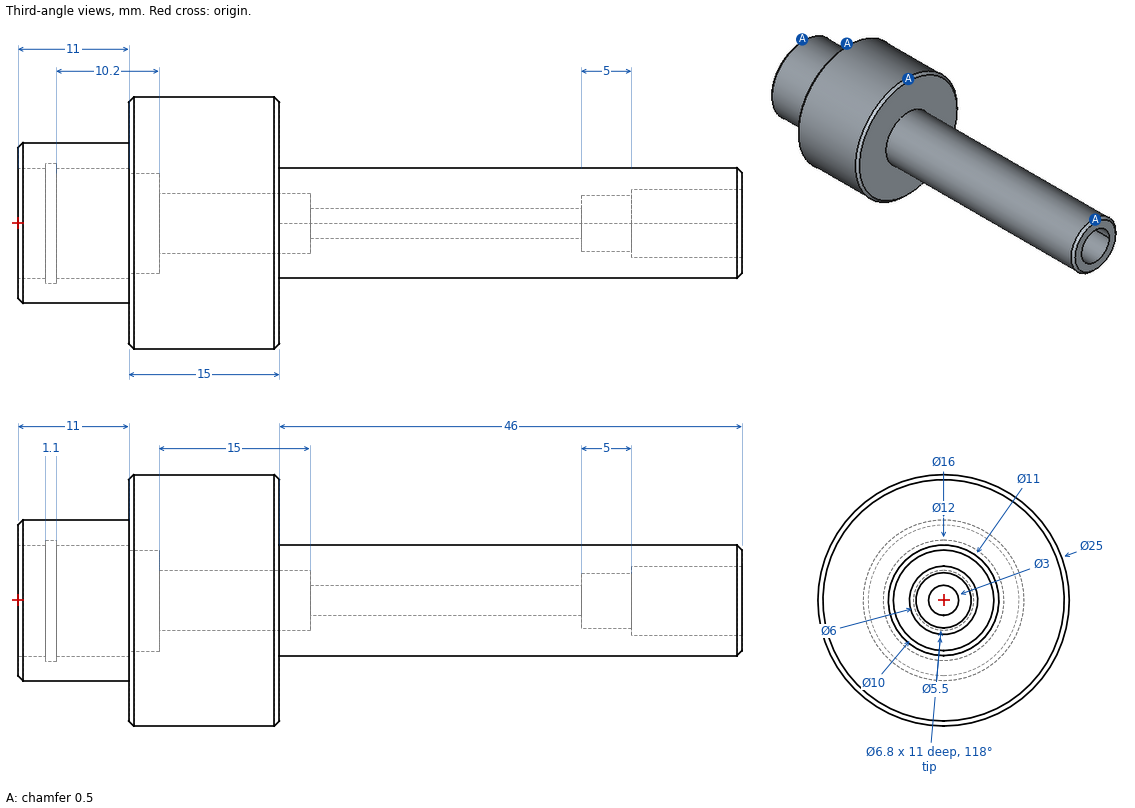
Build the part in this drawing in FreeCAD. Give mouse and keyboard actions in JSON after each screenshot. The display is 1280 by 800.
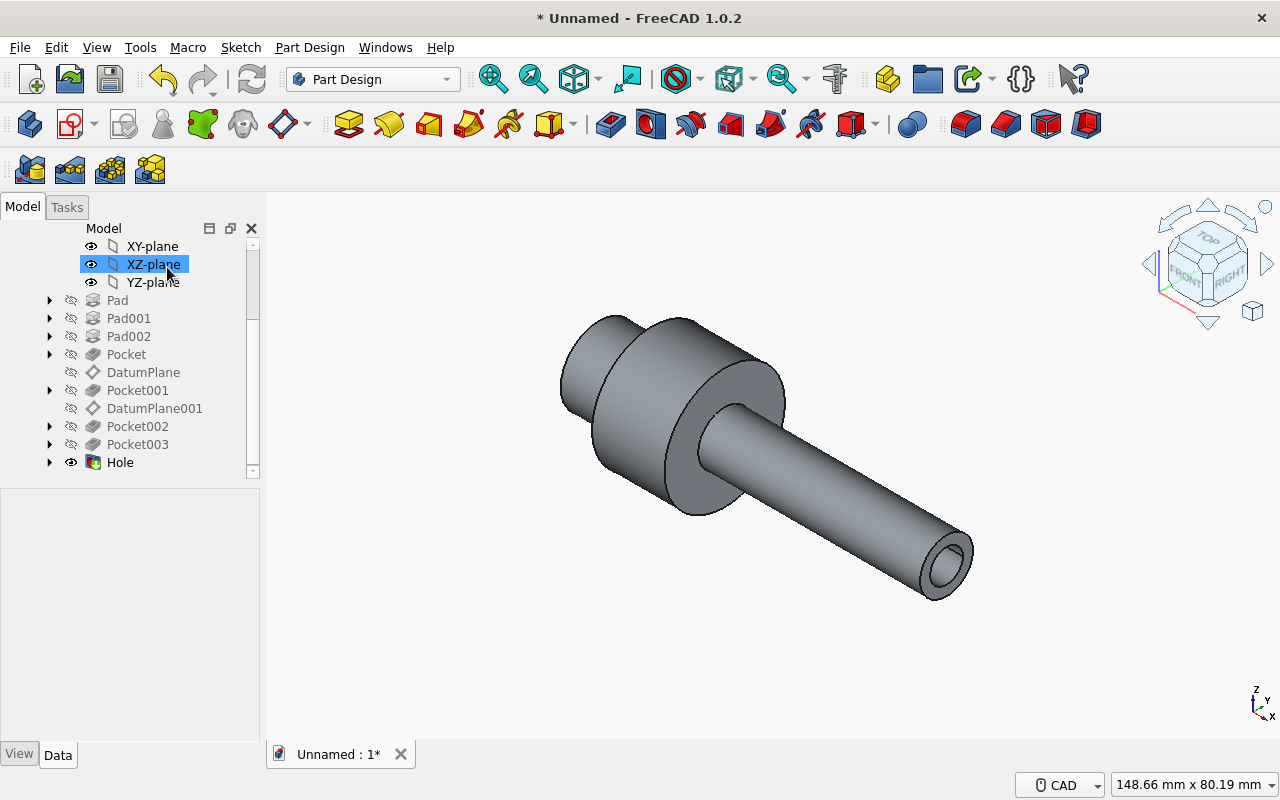
{"action": "scroll", "coordinate": [160, 350], "scroll_direction": "down", "scroll_amount": 3}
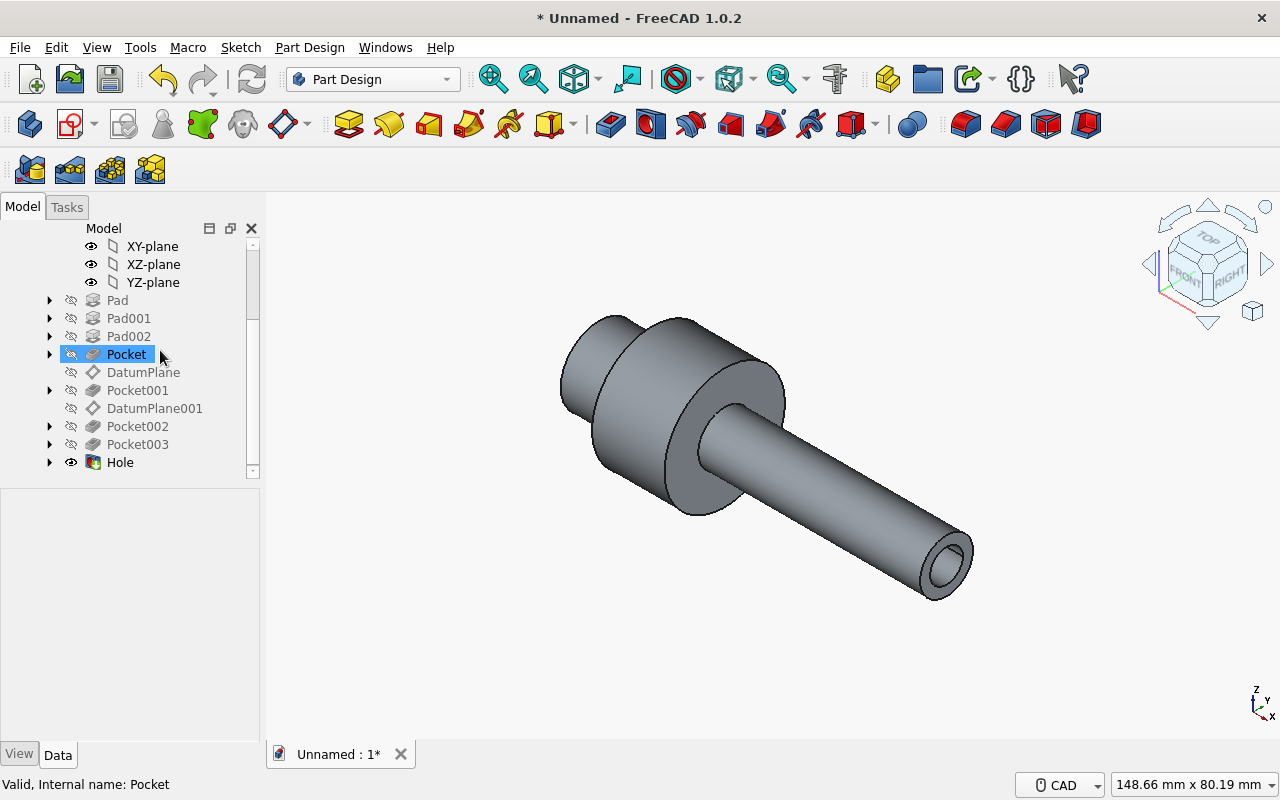
{"action": "scroll", "coordinate": [160, 350], "scroll_direction": "up", "scroll_amount": 15}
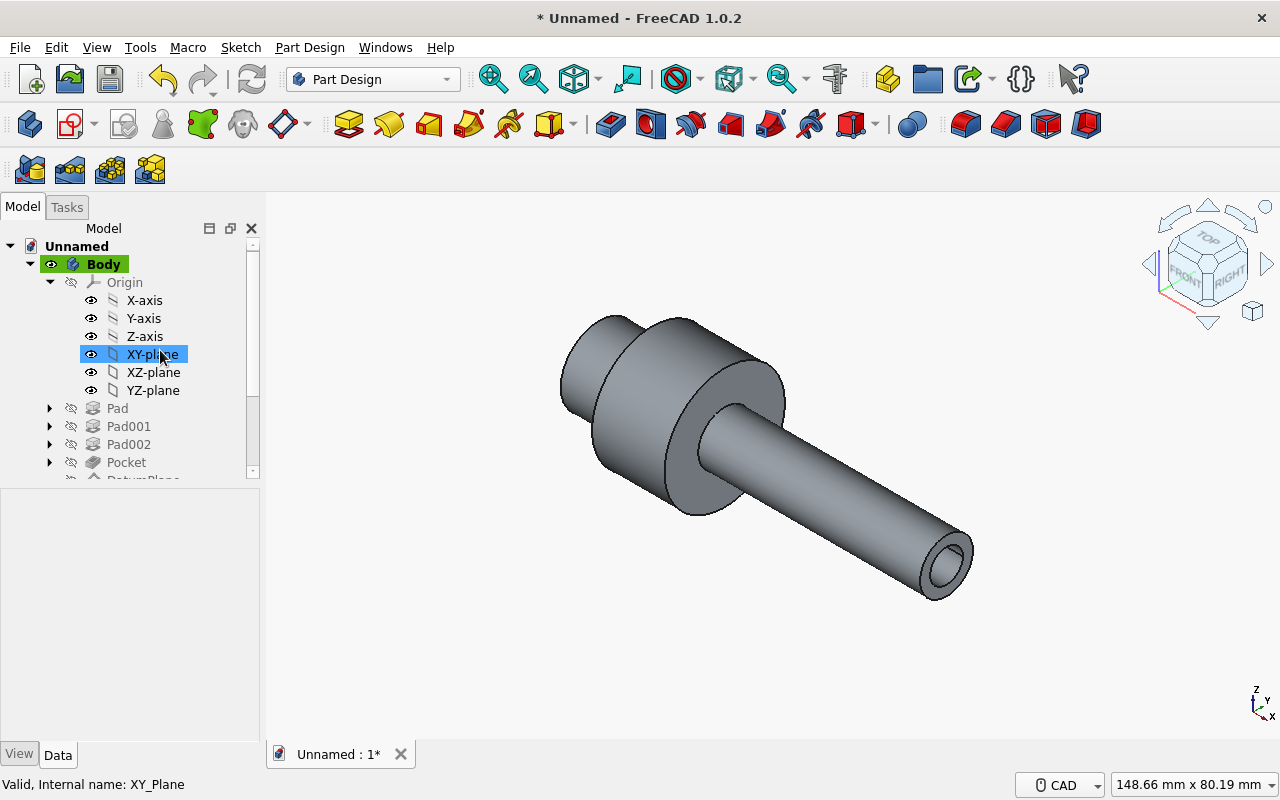
{"action": "left_click", "coordinate": [136, 390]}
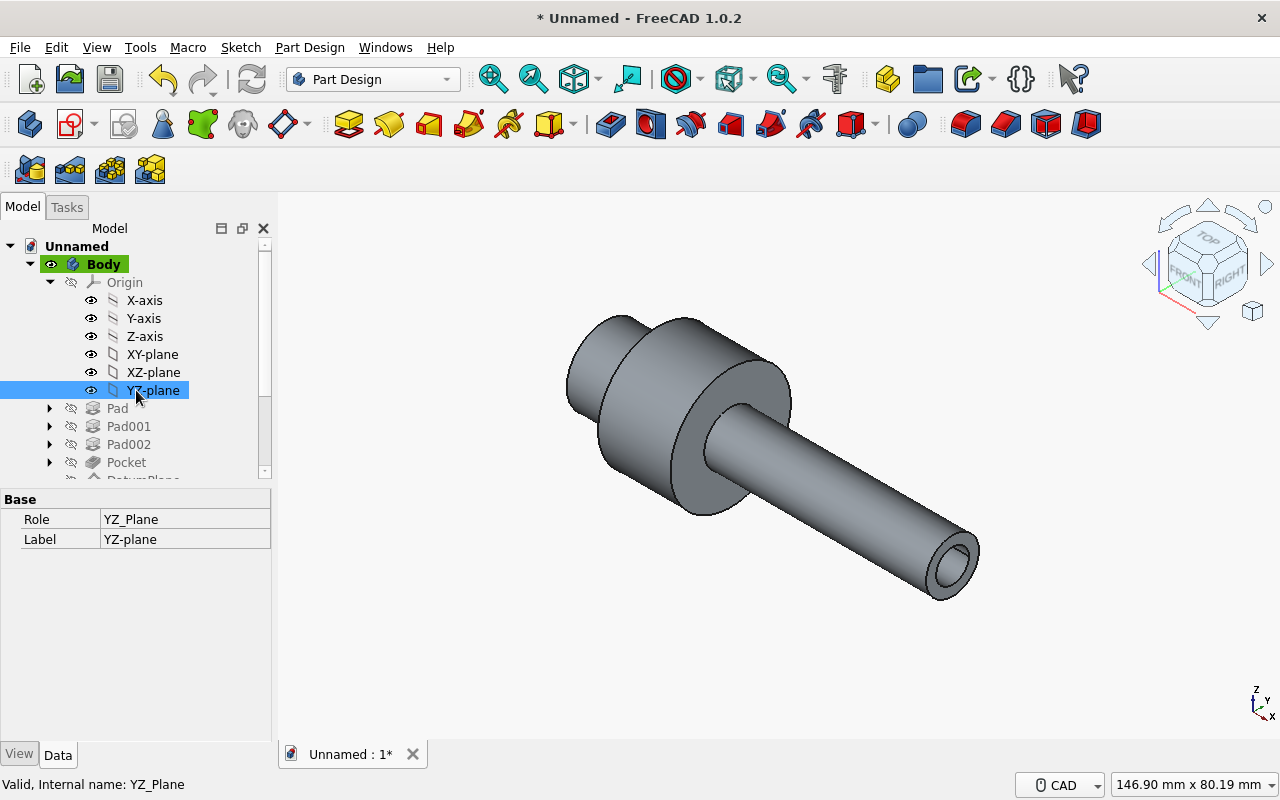
{"action": "left_click", "coordinate": [284, 124]}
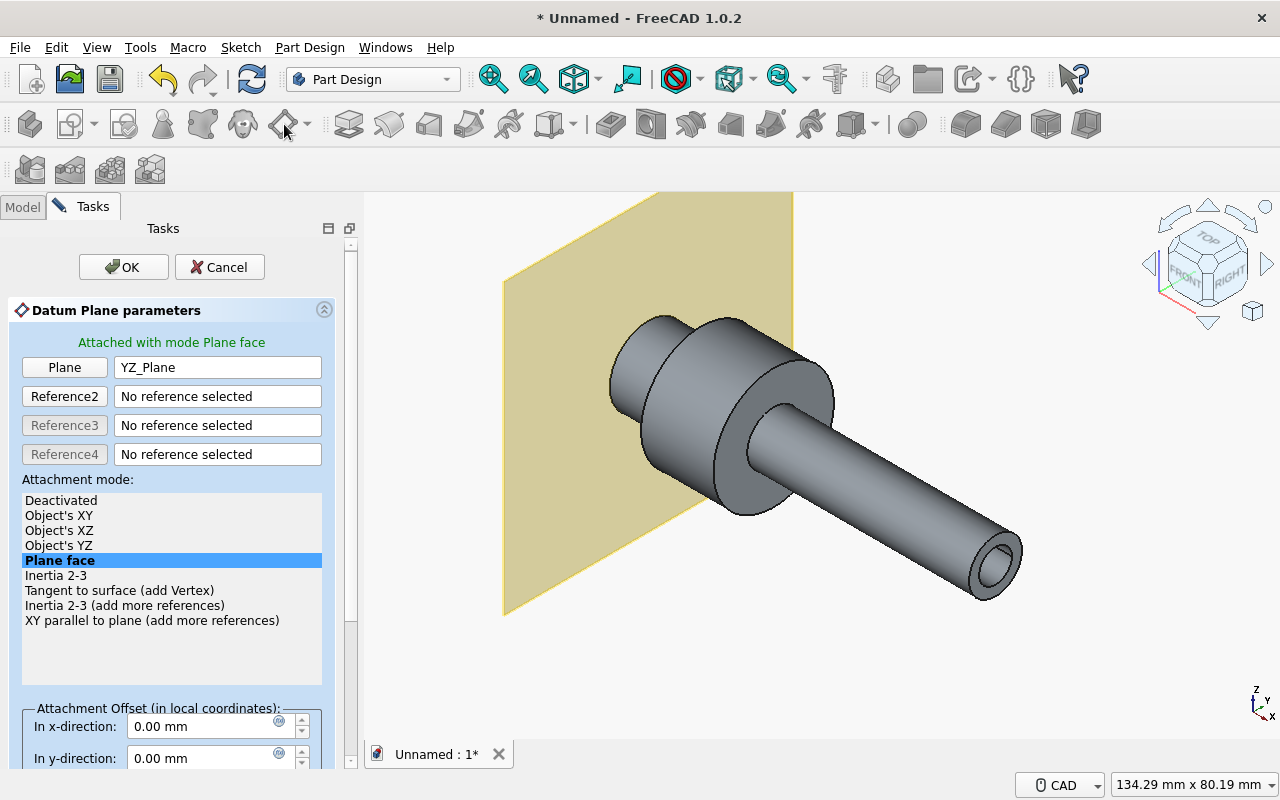
{"action": "scroll", "coordinate": [351, 503], "scroll_direction": "down", "scroll_amount": 2}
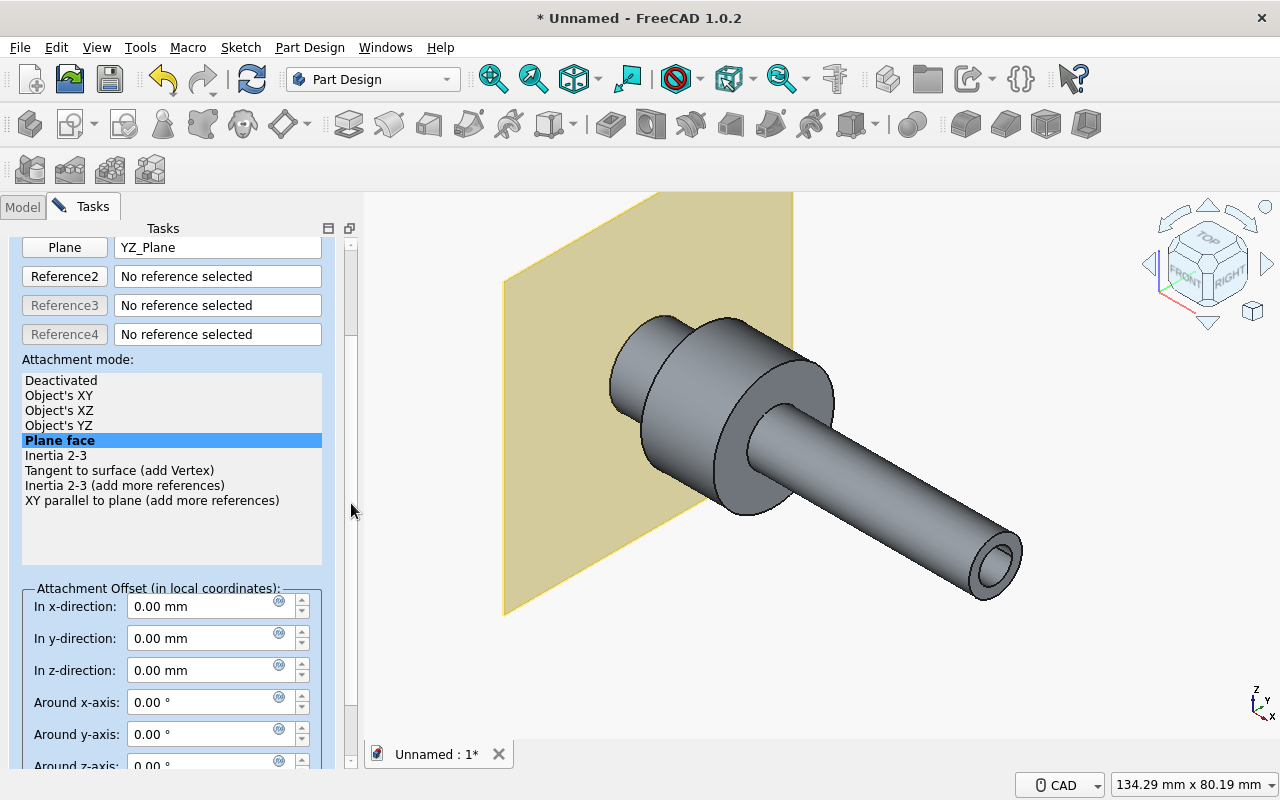
{"action": "triple_click", "coordinate": [210, 670]}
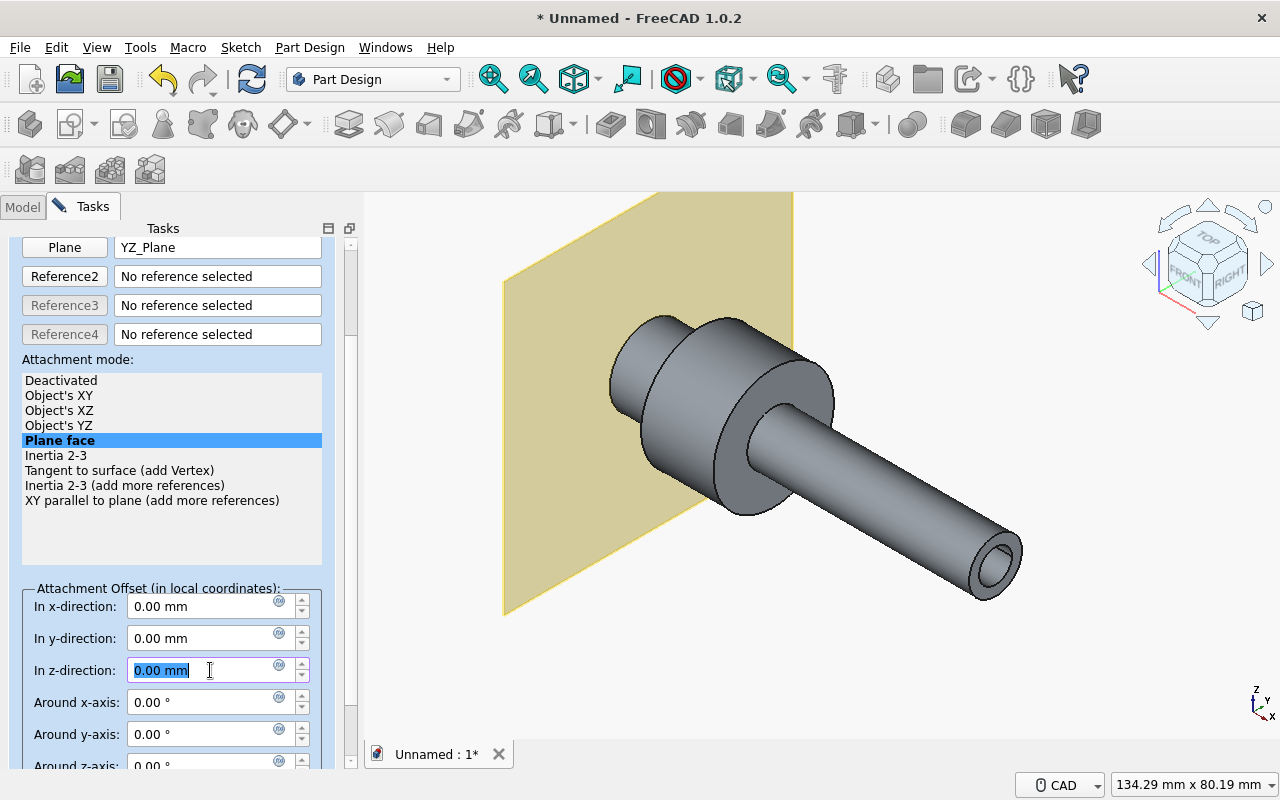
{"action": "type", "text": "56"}
{"action": "key", "text": "Tab"}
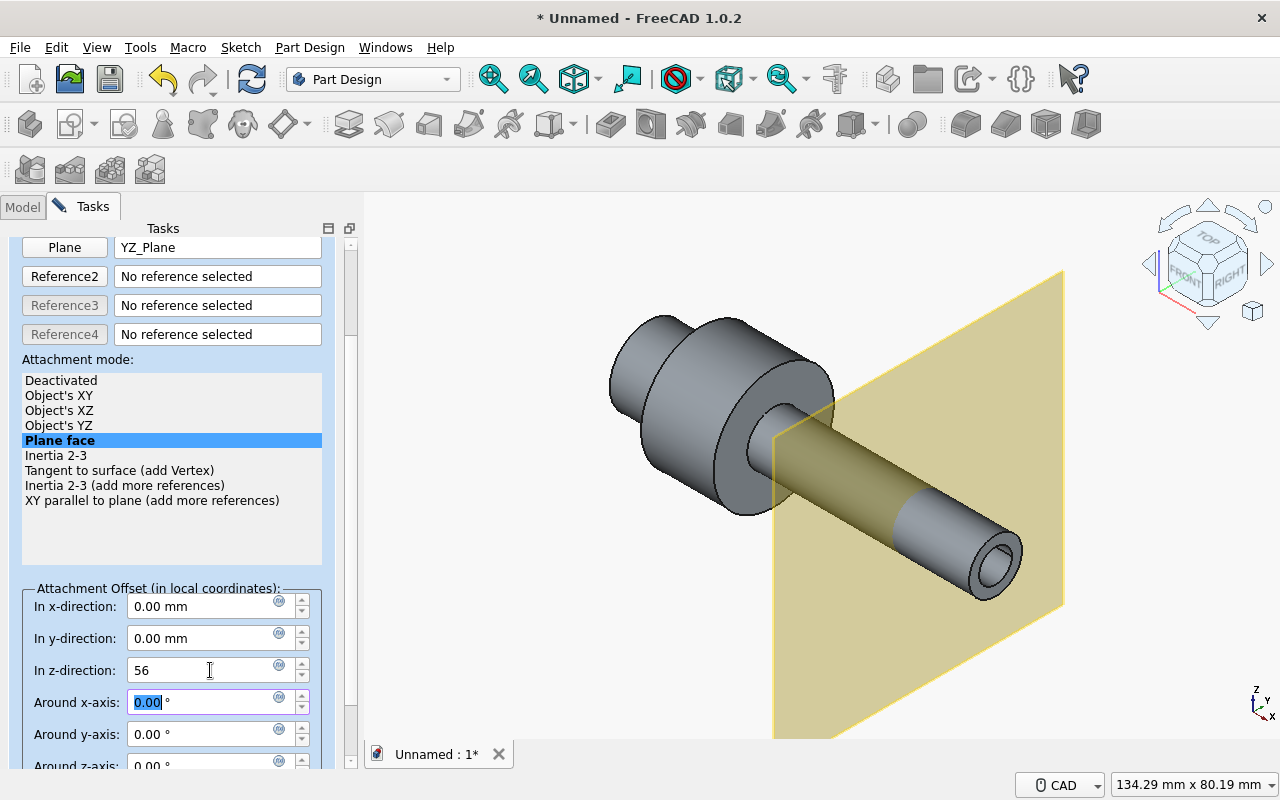
{"action": "scroll", "coordinate": [351, 503], "scroll_direction": "up", "scroll_amount": 3}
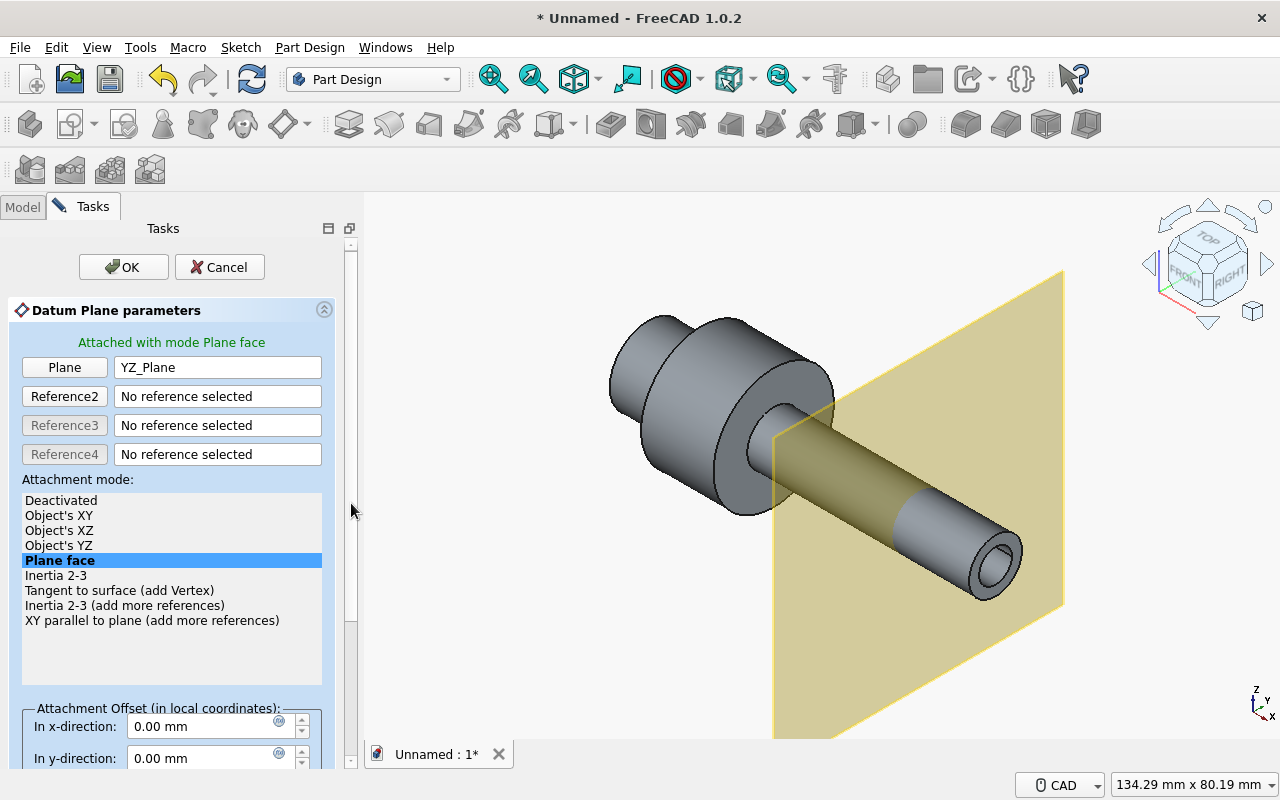
{"action": "left_click", "coordinate": [124, 267]}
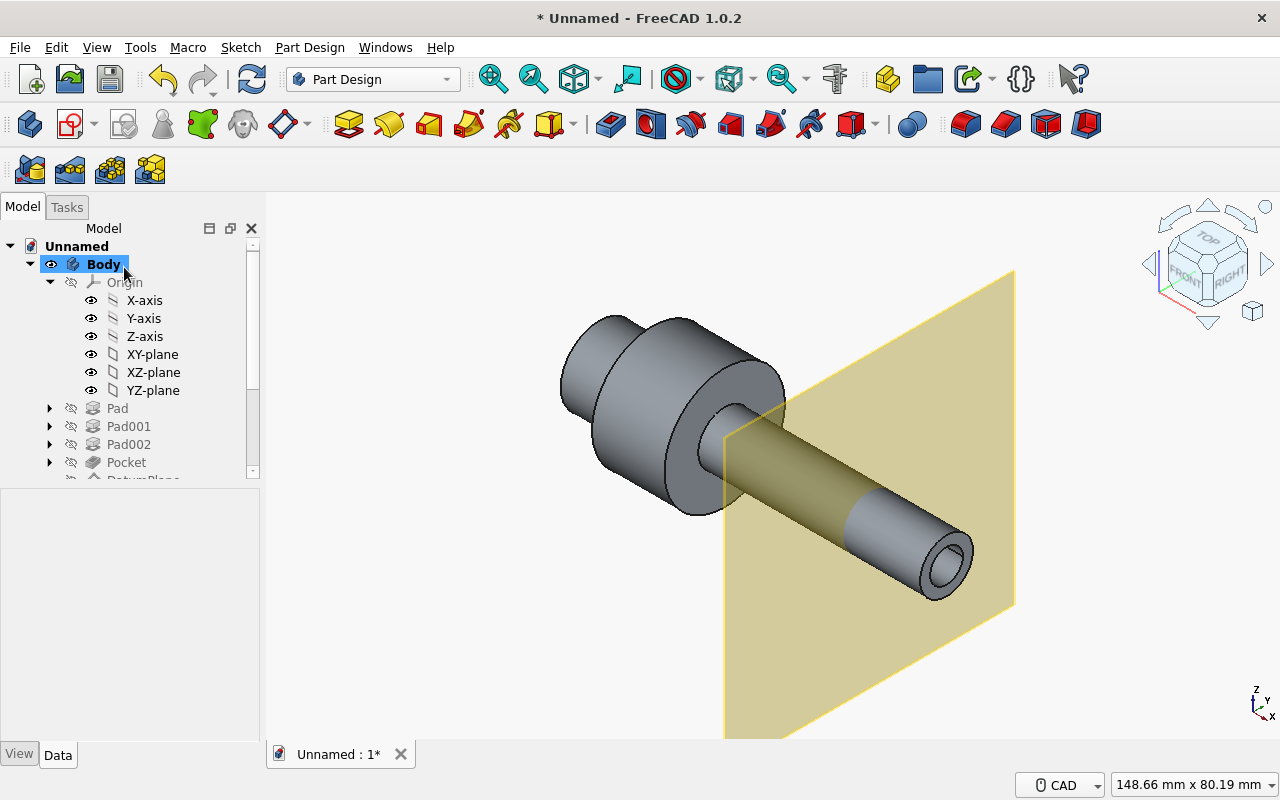
{"action": "scroll", "coordinate": [100, 350], "scroll_direction": "down", "scroll_amount": 3}